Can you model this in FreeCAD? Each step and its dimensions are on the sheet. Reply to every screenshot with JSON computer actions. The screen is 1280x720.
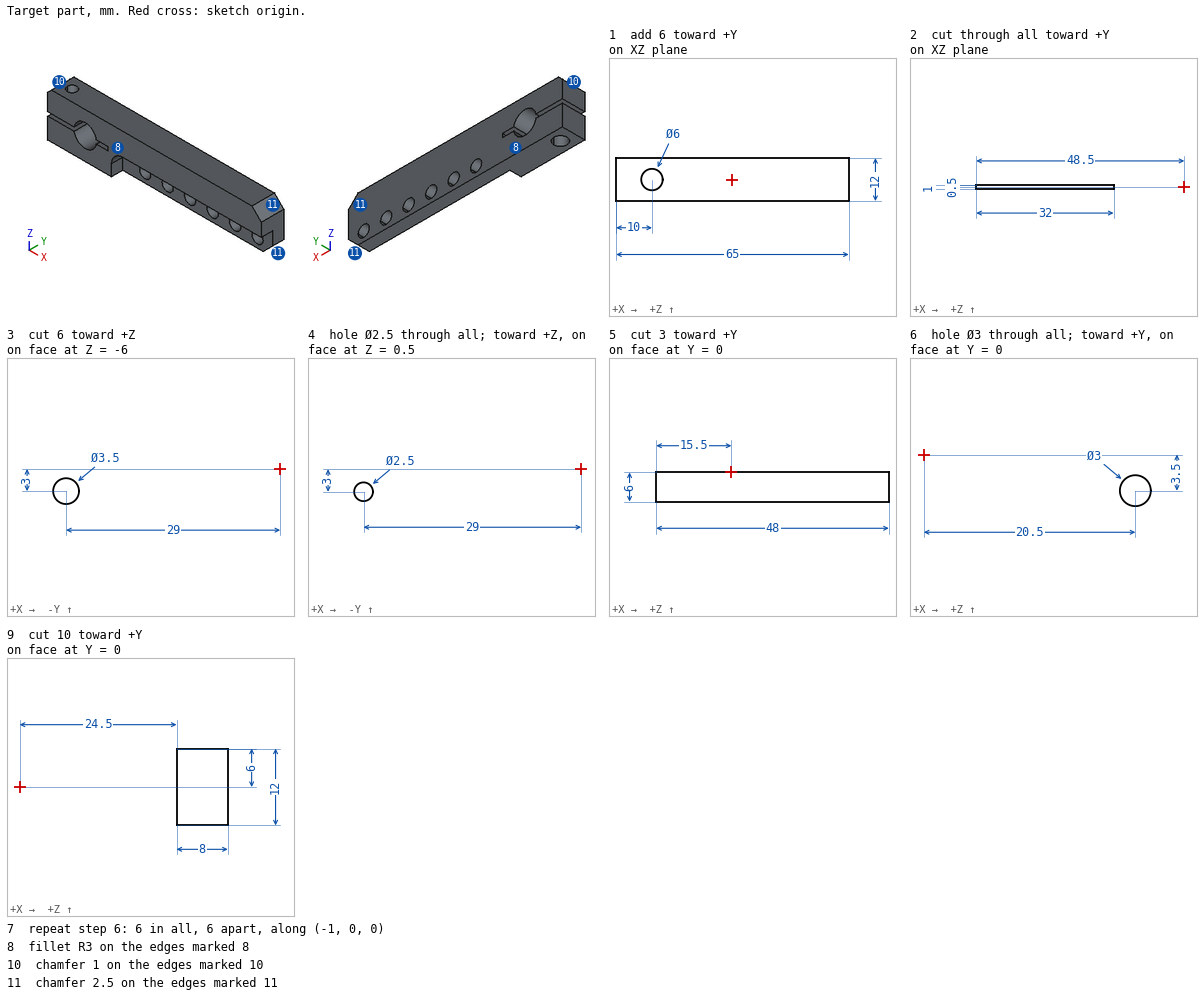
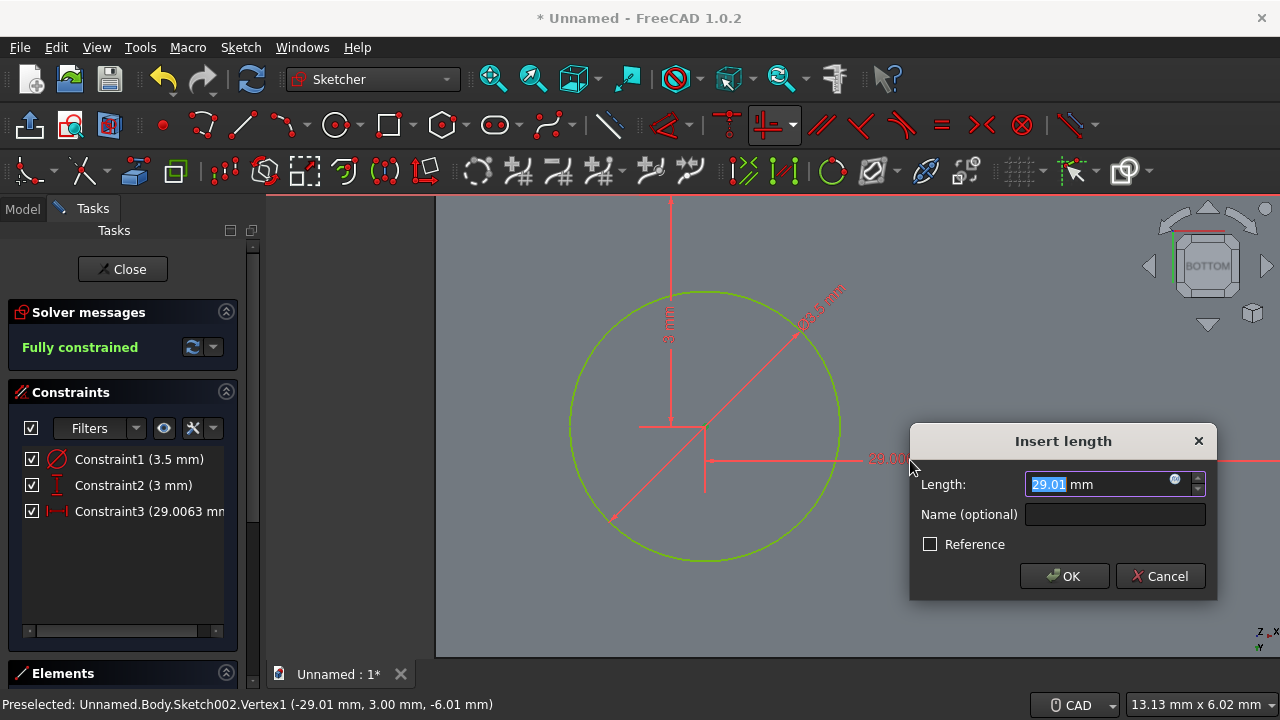
{"action": "type", "text": "29"}
{"action": "key", "text": "Return"}
{"action": "key", "text": "Escape"}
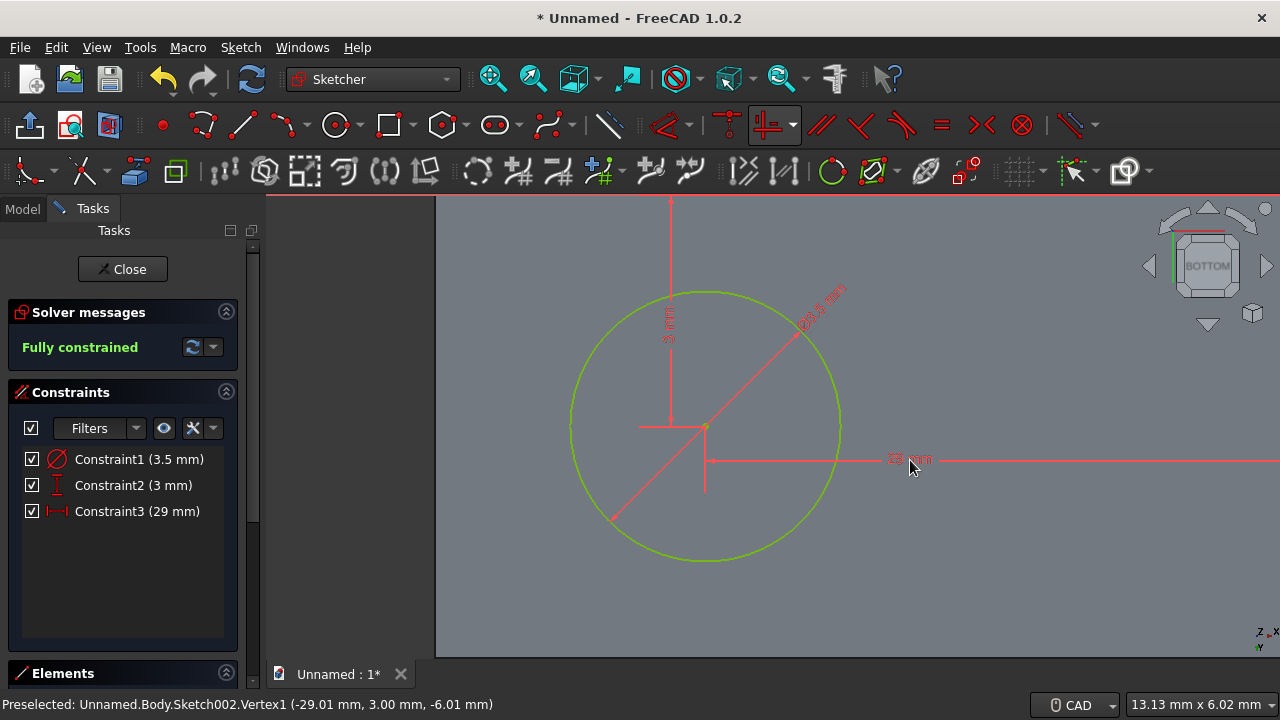
{"action": "left_click", "coordinate": [123, 269]}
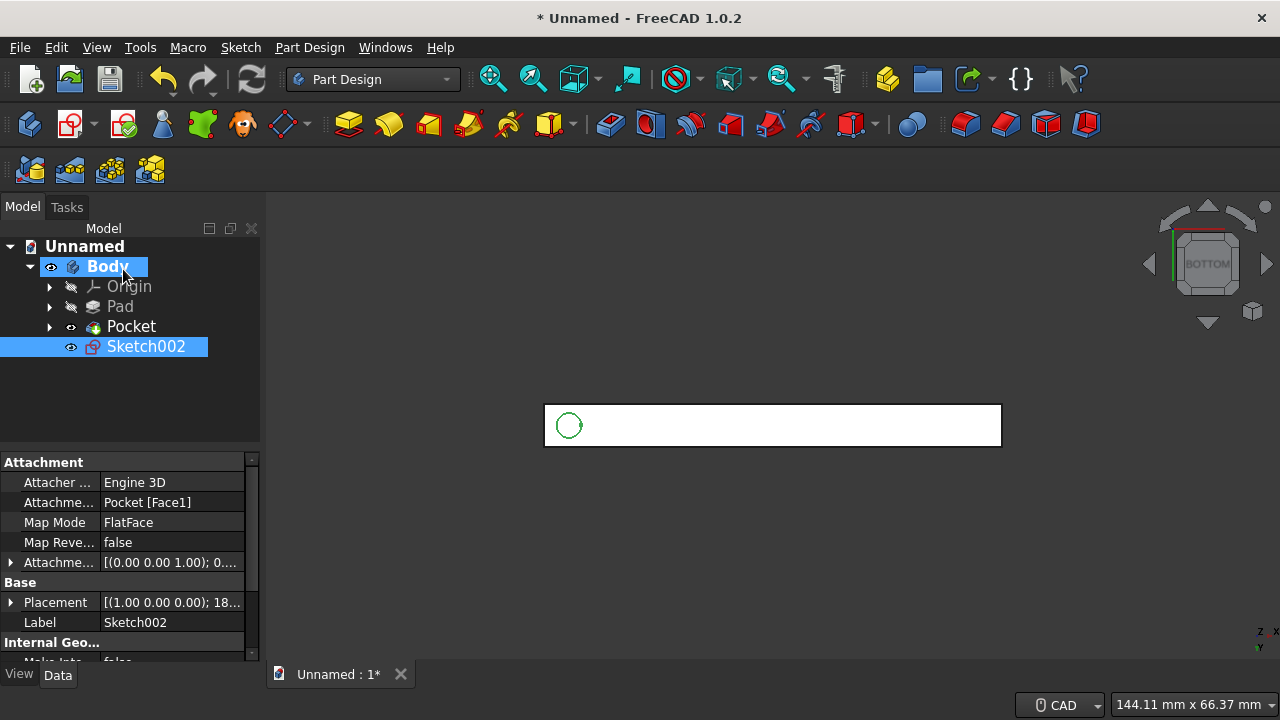
{"action": "left_click", "coordinate": [612, 124]}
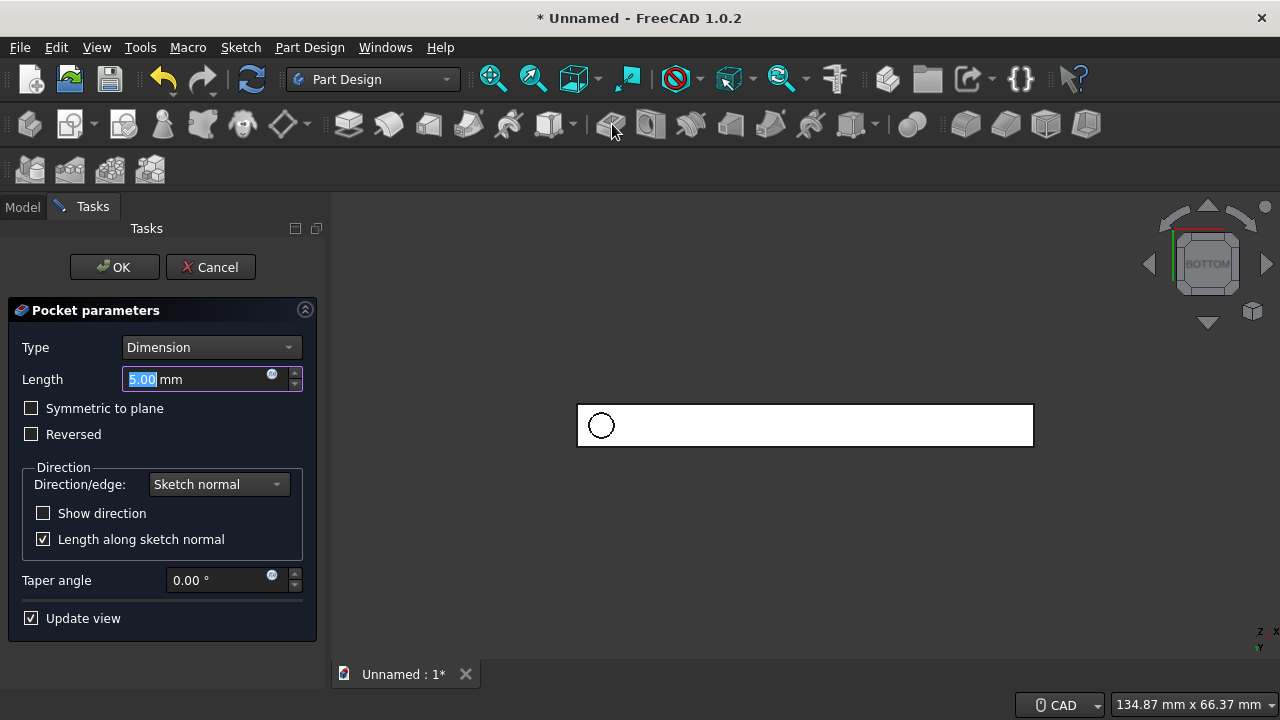
{"action": "type", "text": "6"}
{"action": "key", "text": "Tab"}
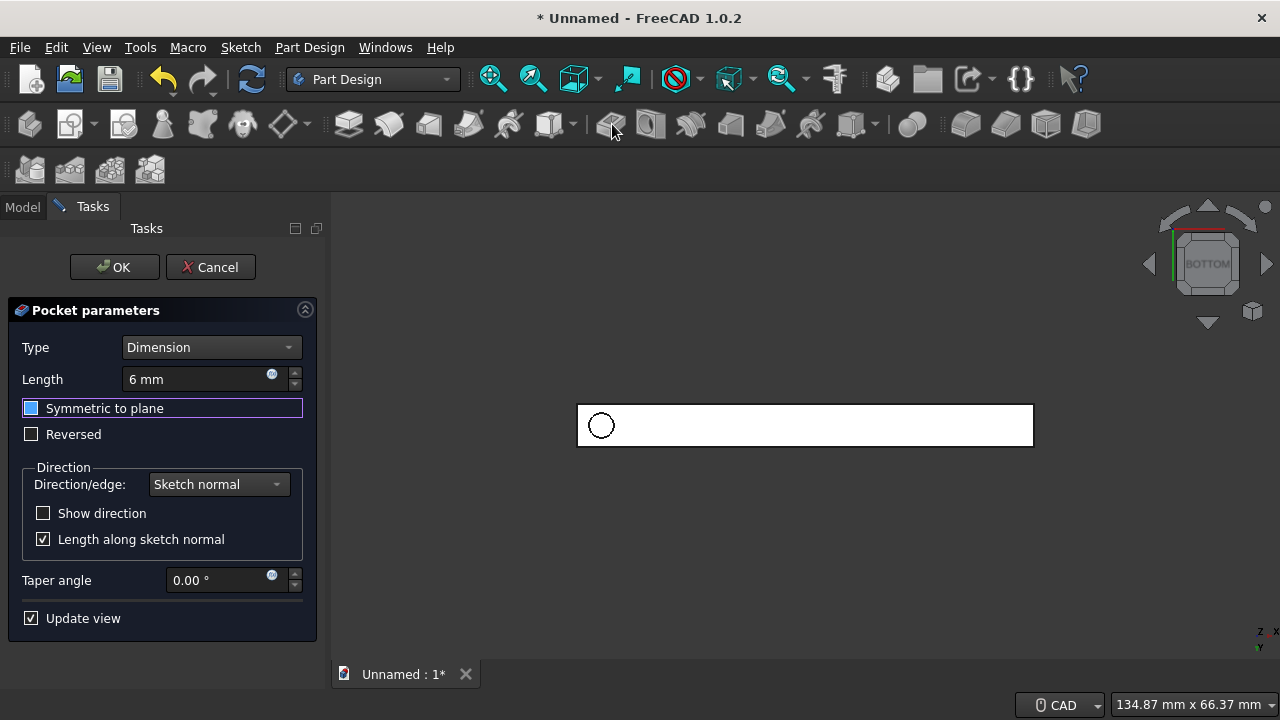
{"action": "left_click", "coordinate": [115, 267]}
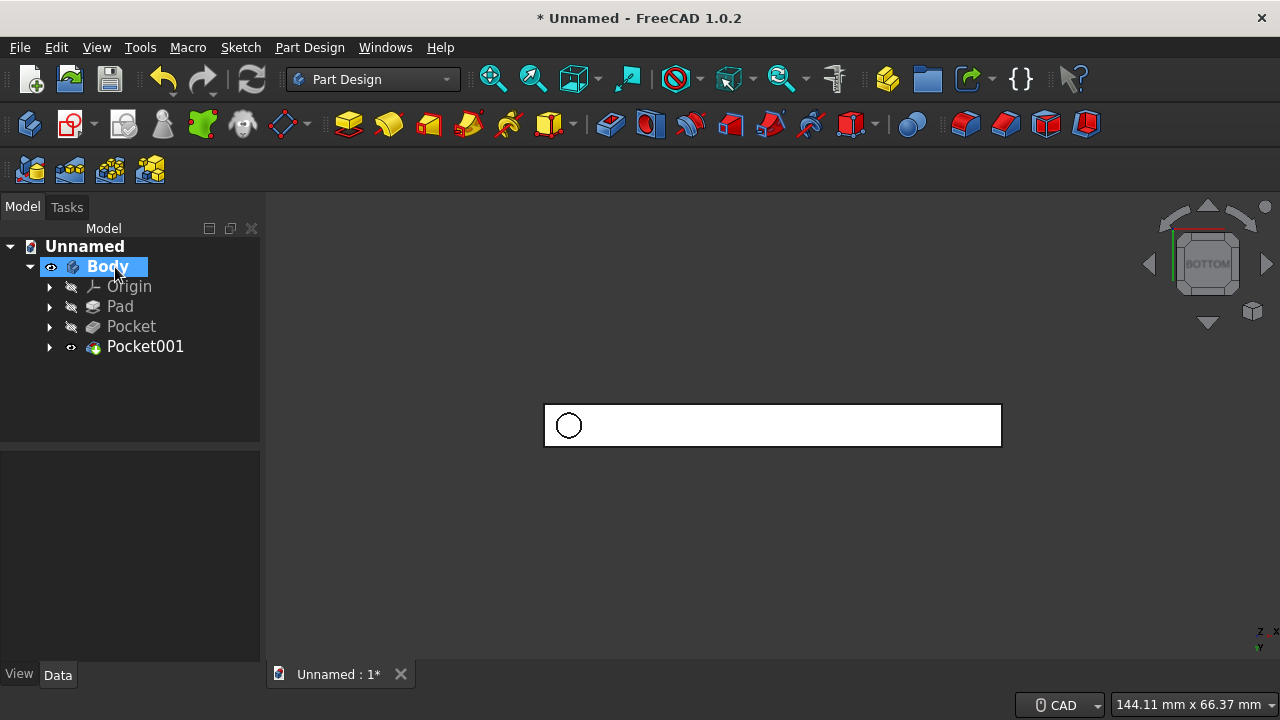
{"action": "left_click", "coordinate": [569, 425]}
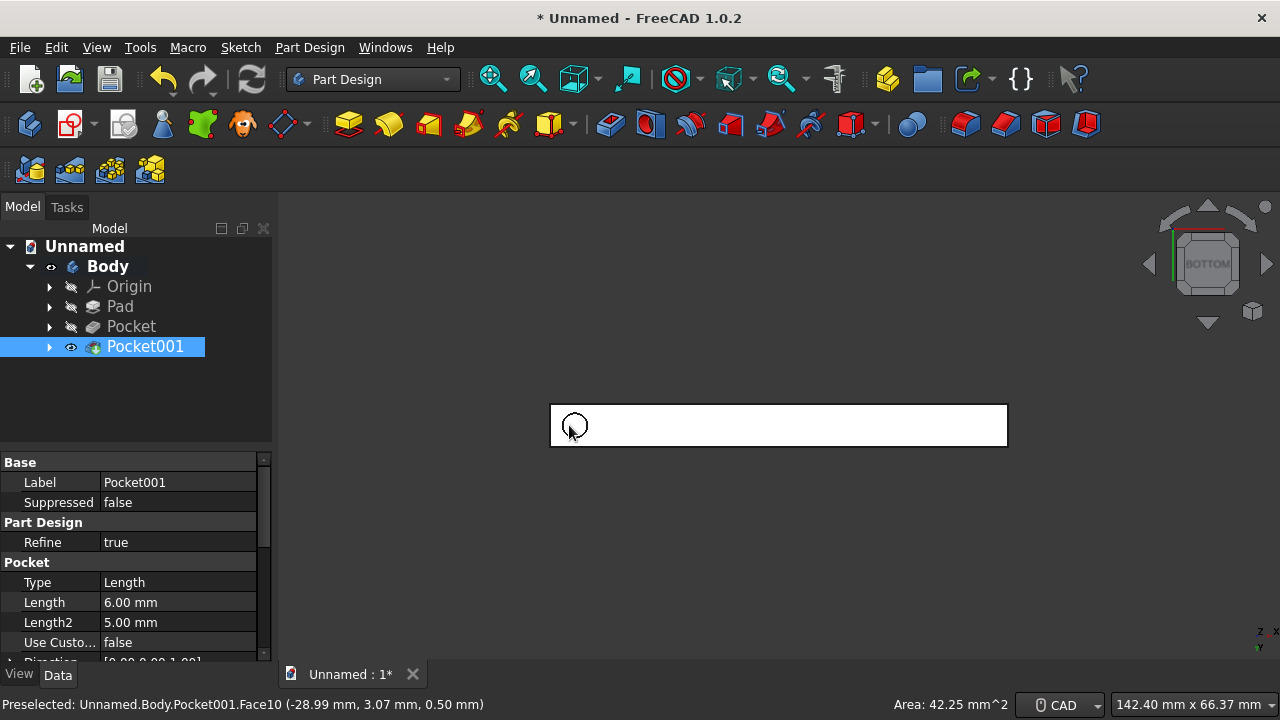
{"action": "left_click", "coordinate": [70, 124]}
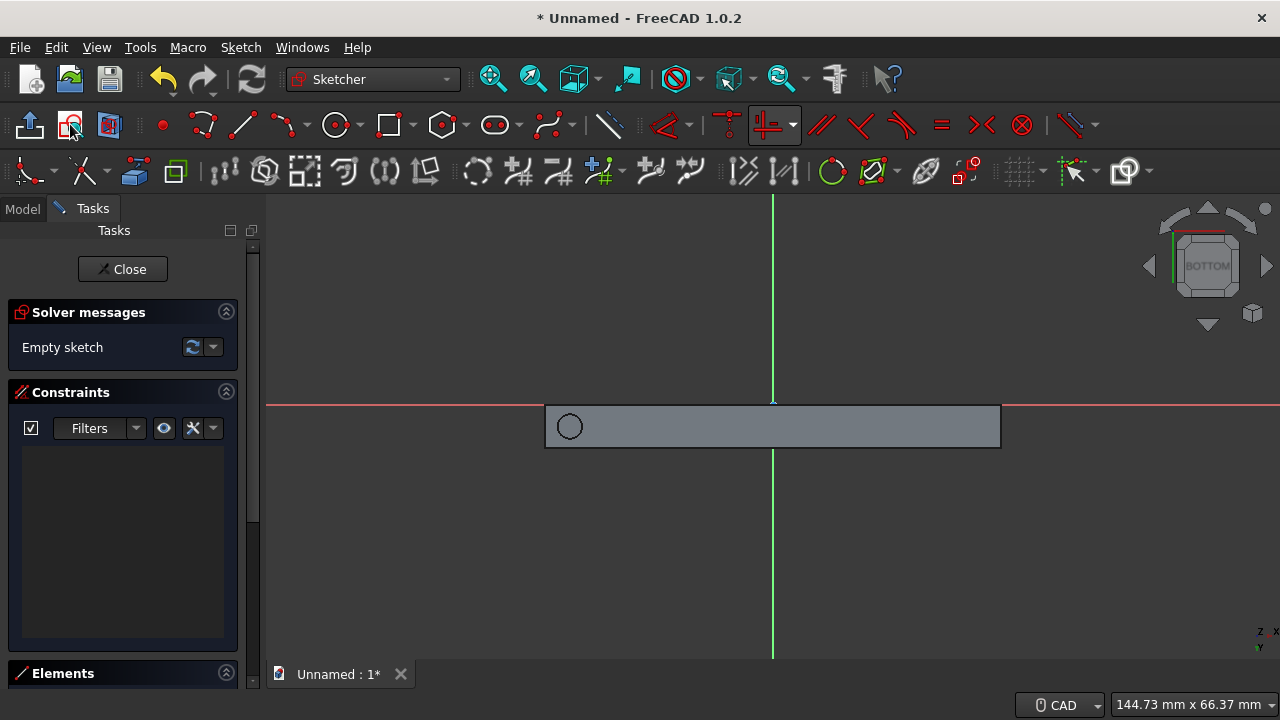
{"action": "left_click", "coordinate": [110, 126]}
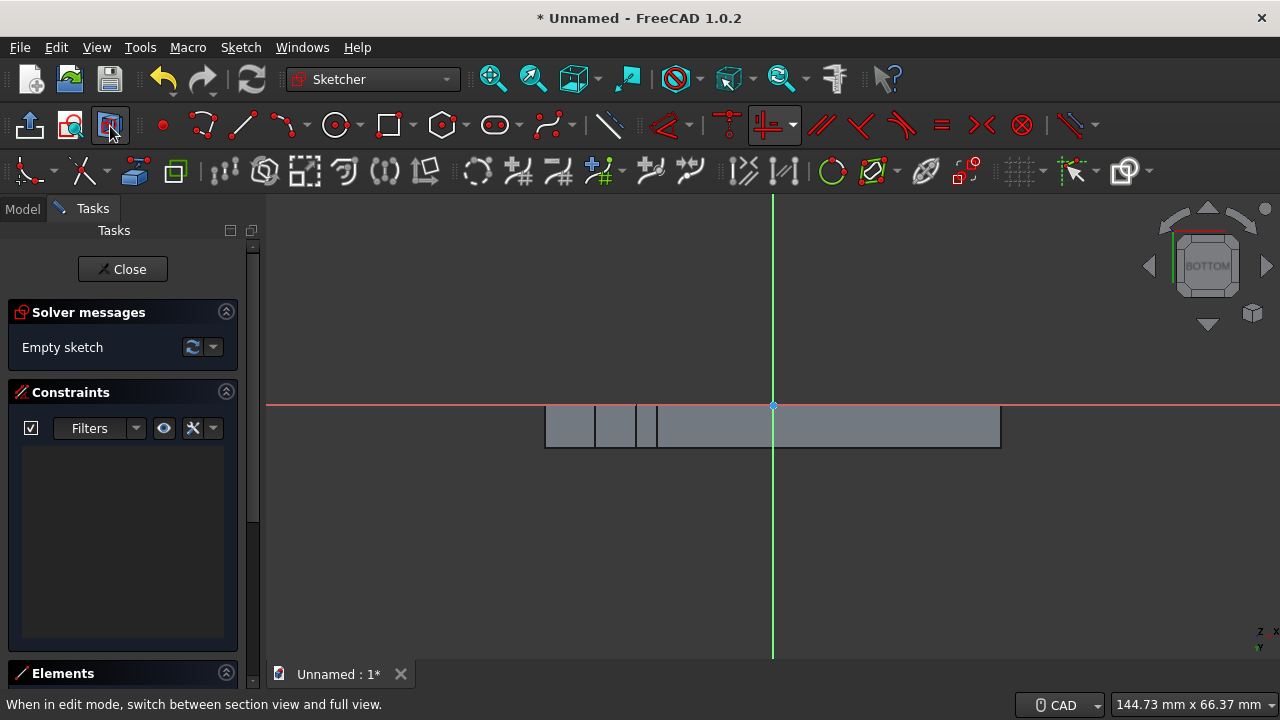
{"action": "scroll", "coordinate": [561, 427], "scroll_direction": "up", "scroll_amount": 14}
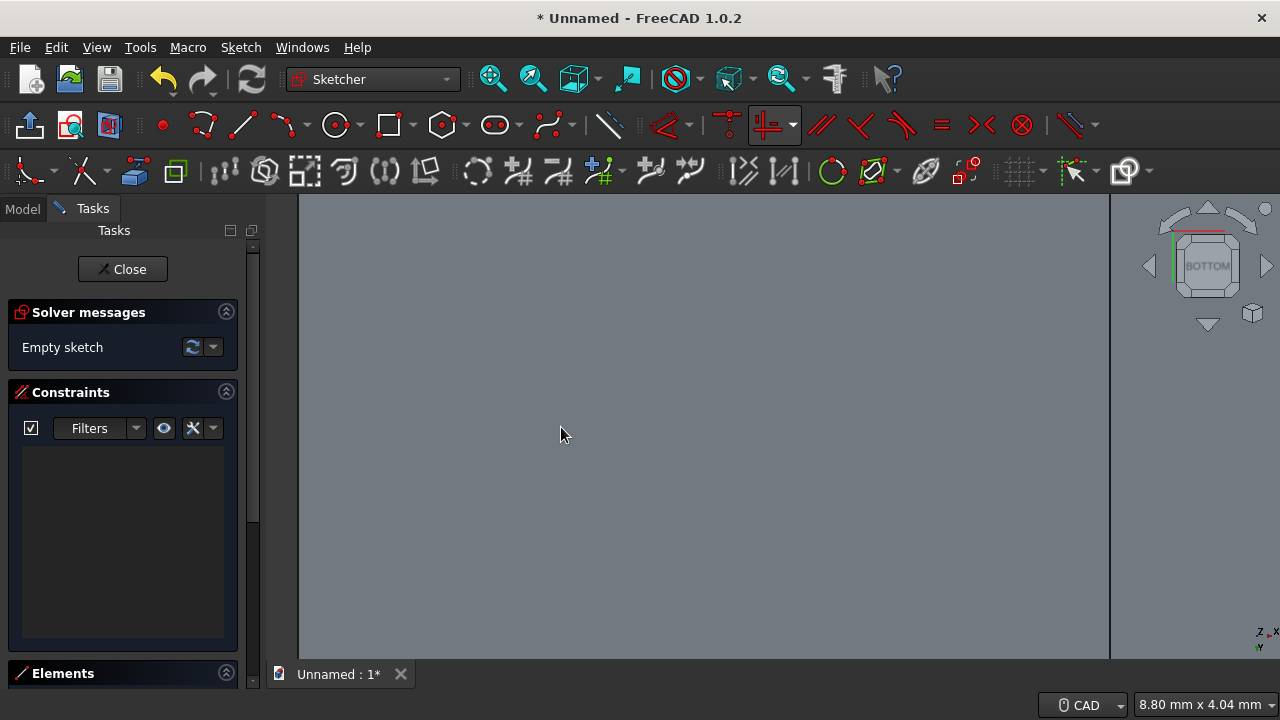
{"action": "key", "text": "g c"}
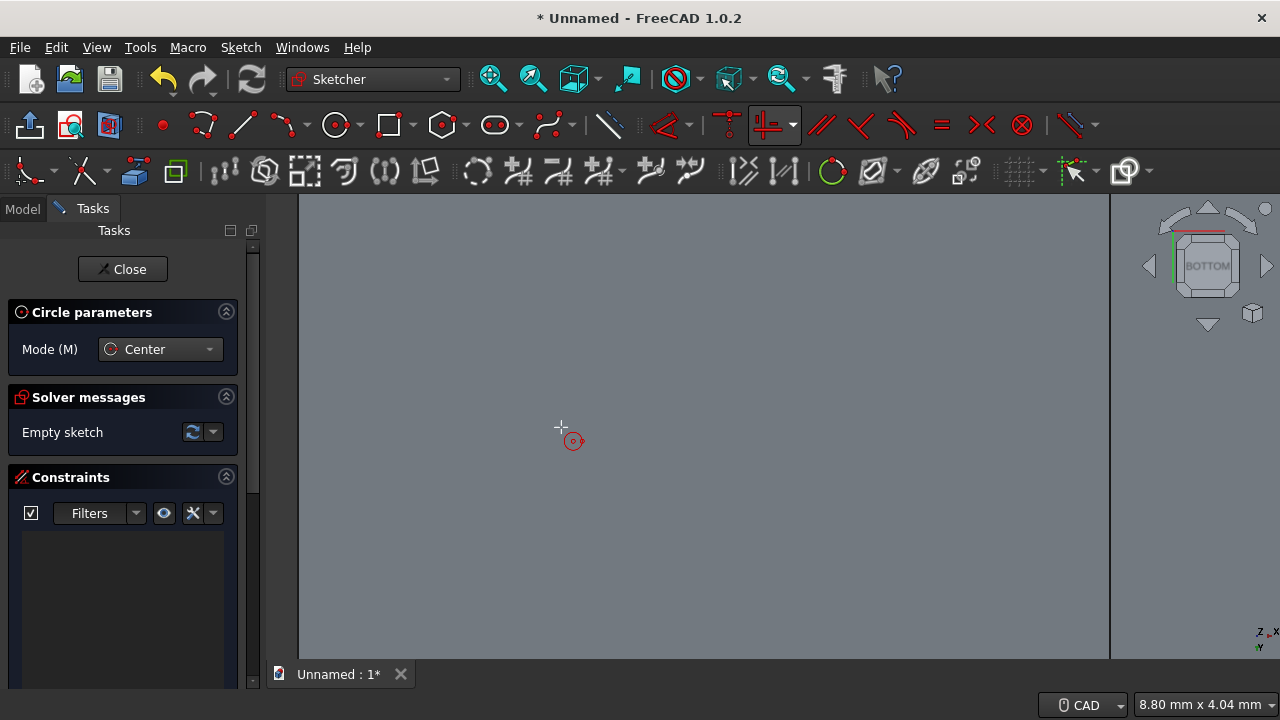
{"action": "left_click", "coordinate": [702, 411]}
{"action": "left_click", "coordinate": [803, 309]}
{"action": "key", "text": "Escape"}